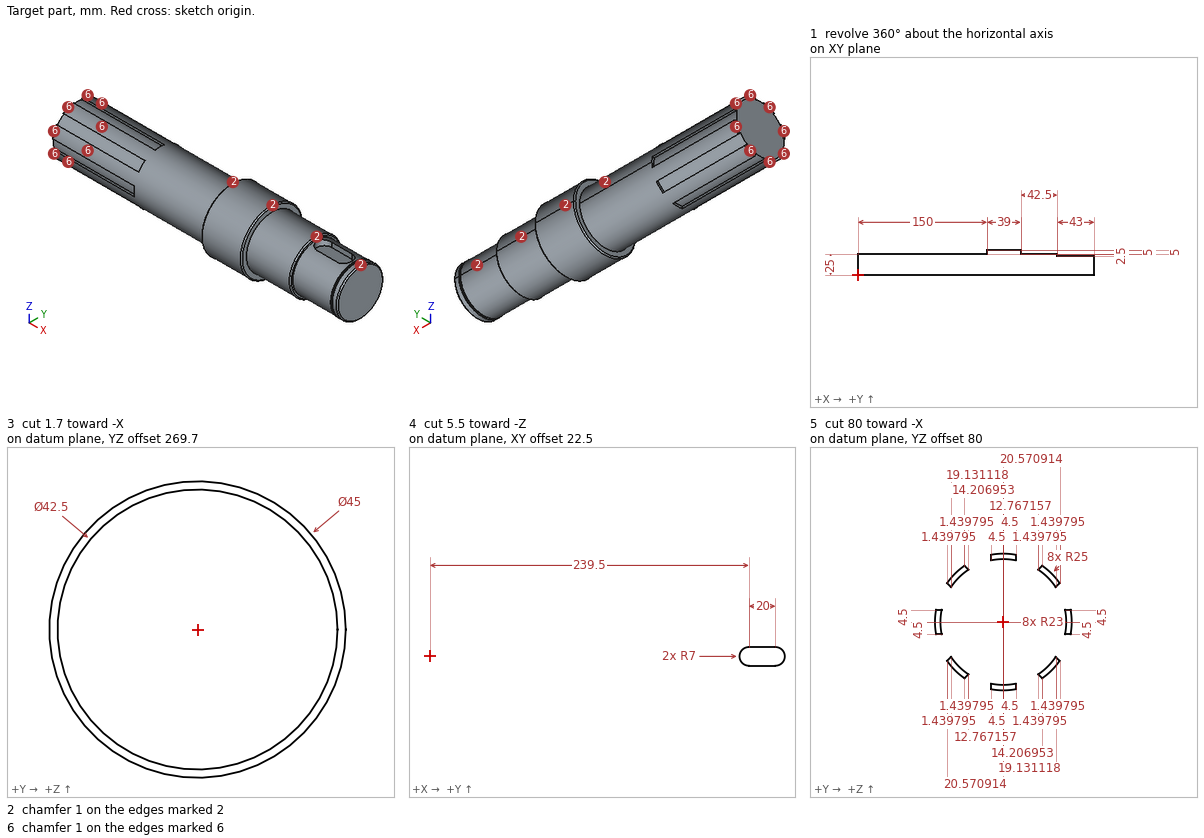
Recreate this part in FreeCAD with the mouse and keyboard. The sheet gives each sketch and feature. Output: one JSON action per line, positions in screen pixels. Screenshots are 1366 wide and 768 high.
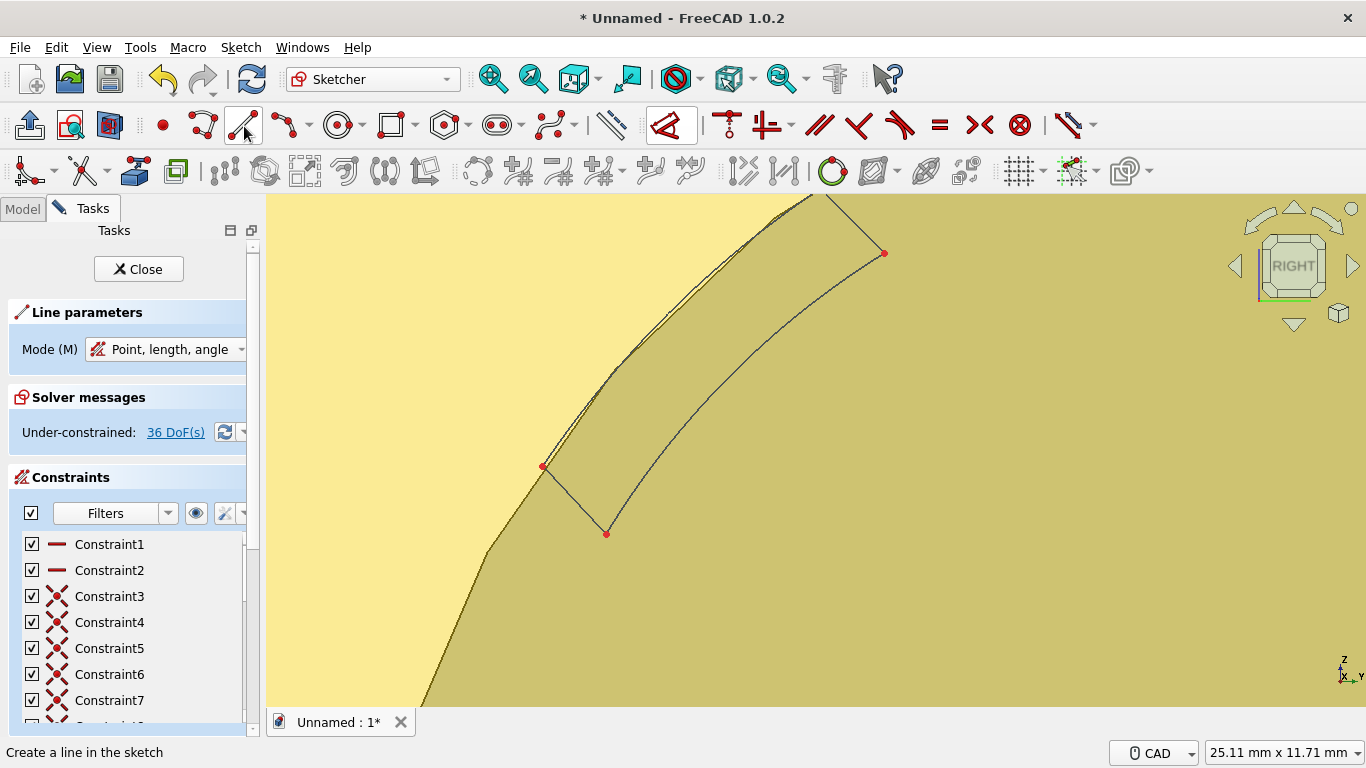
{"action": "scroll", "coordinate": [638, 351], "scroll_direction": "down", "scroll_amount": 10}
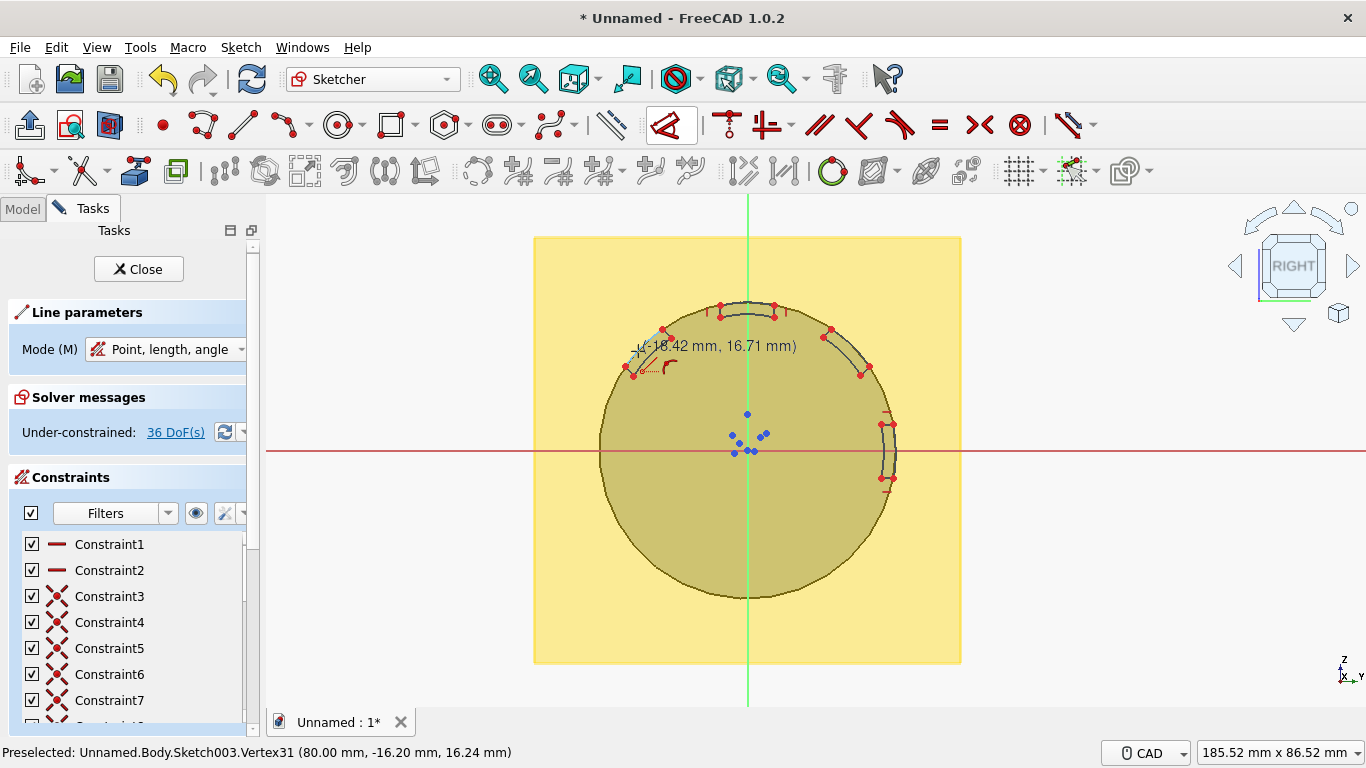
{"action": "left_click", "coordinate": [614, 477]}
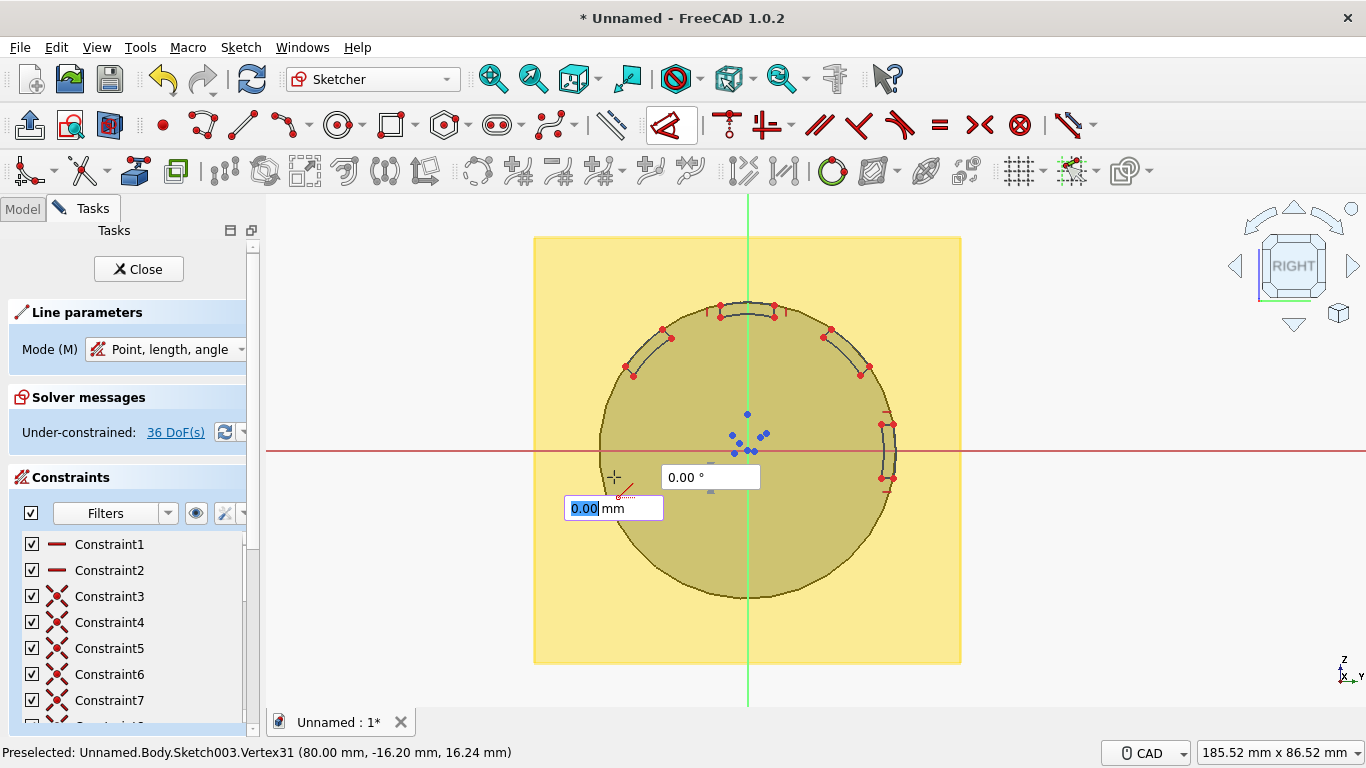
{"action": "scroll", "coordinate": [602, 477], "scroll_direction": "up", "scroll_amount": 2}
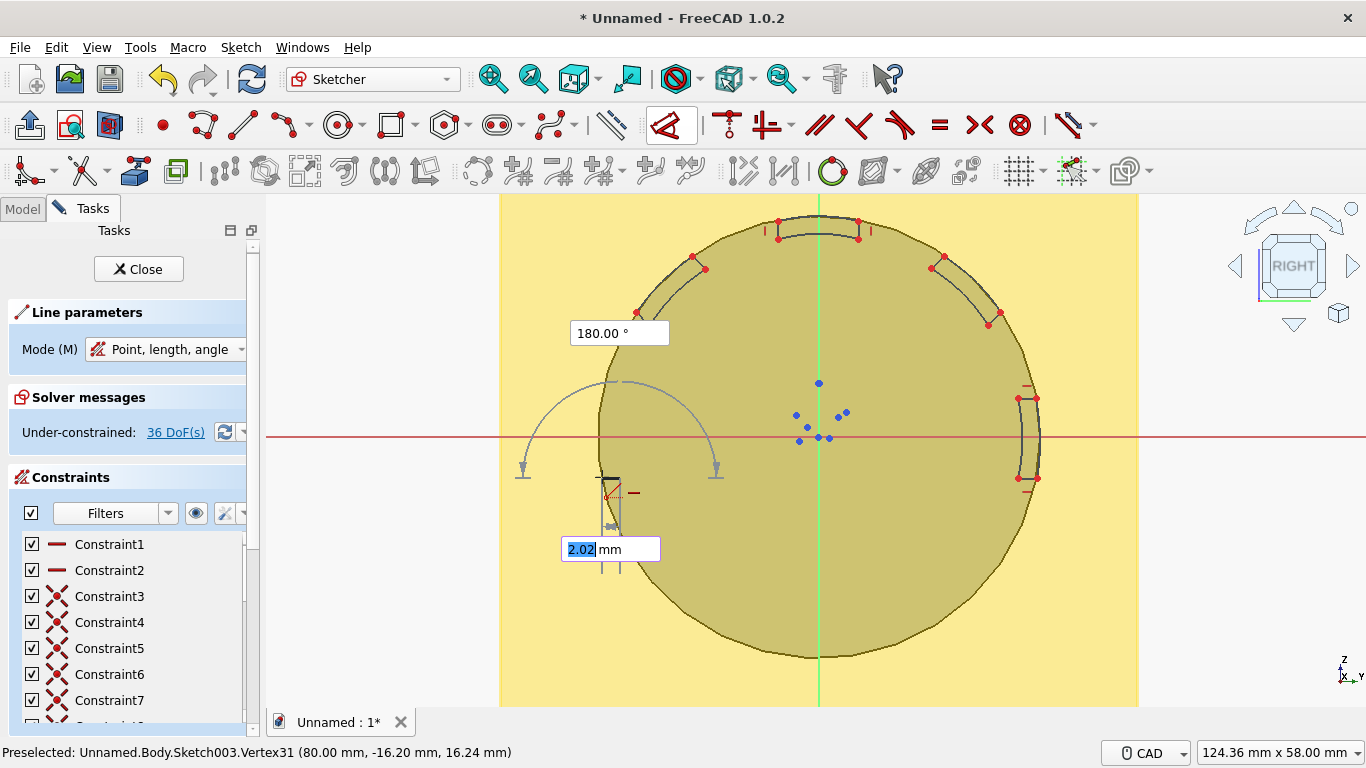
{"action": "left_click", "coordinate": [601, 477]}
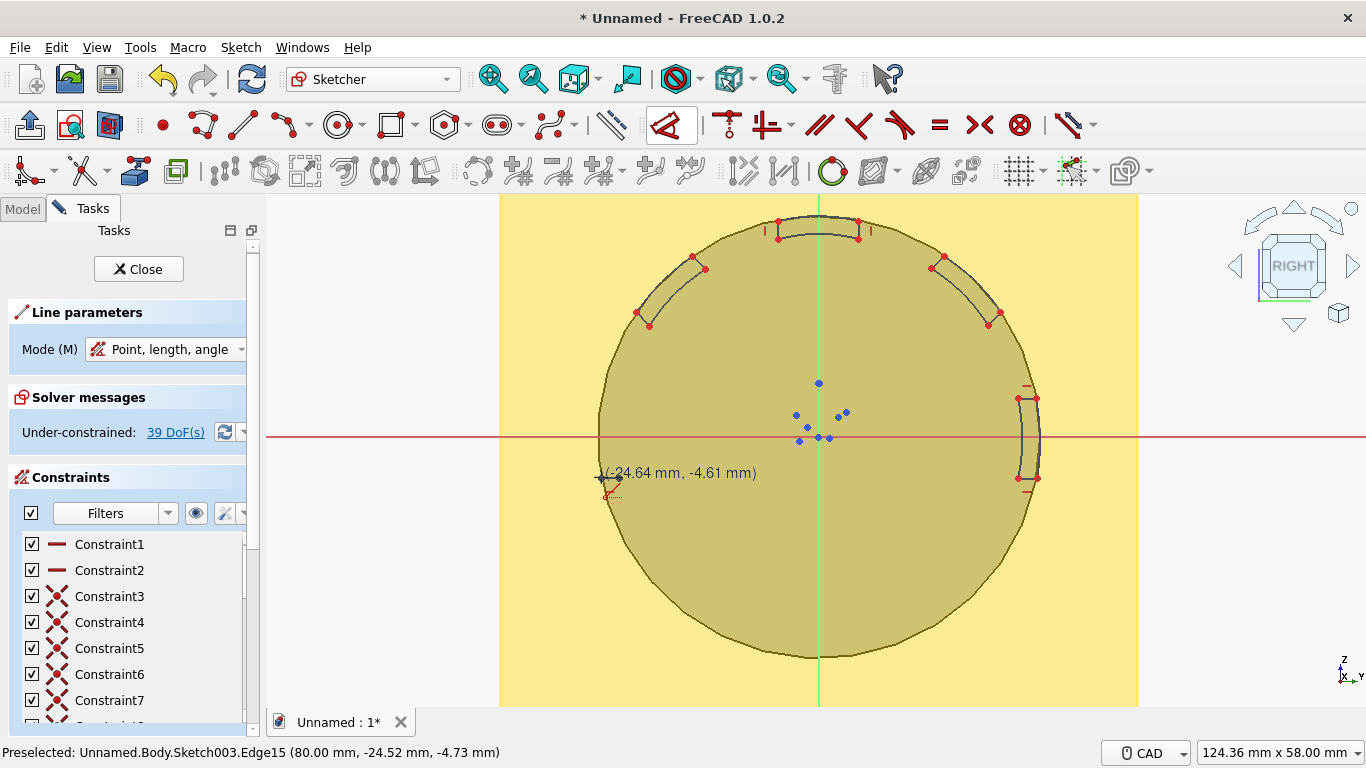
{"action": "left_click", "coordinate": [601, 397]}
{"action": "left_click", "coordinate": [619, 397]}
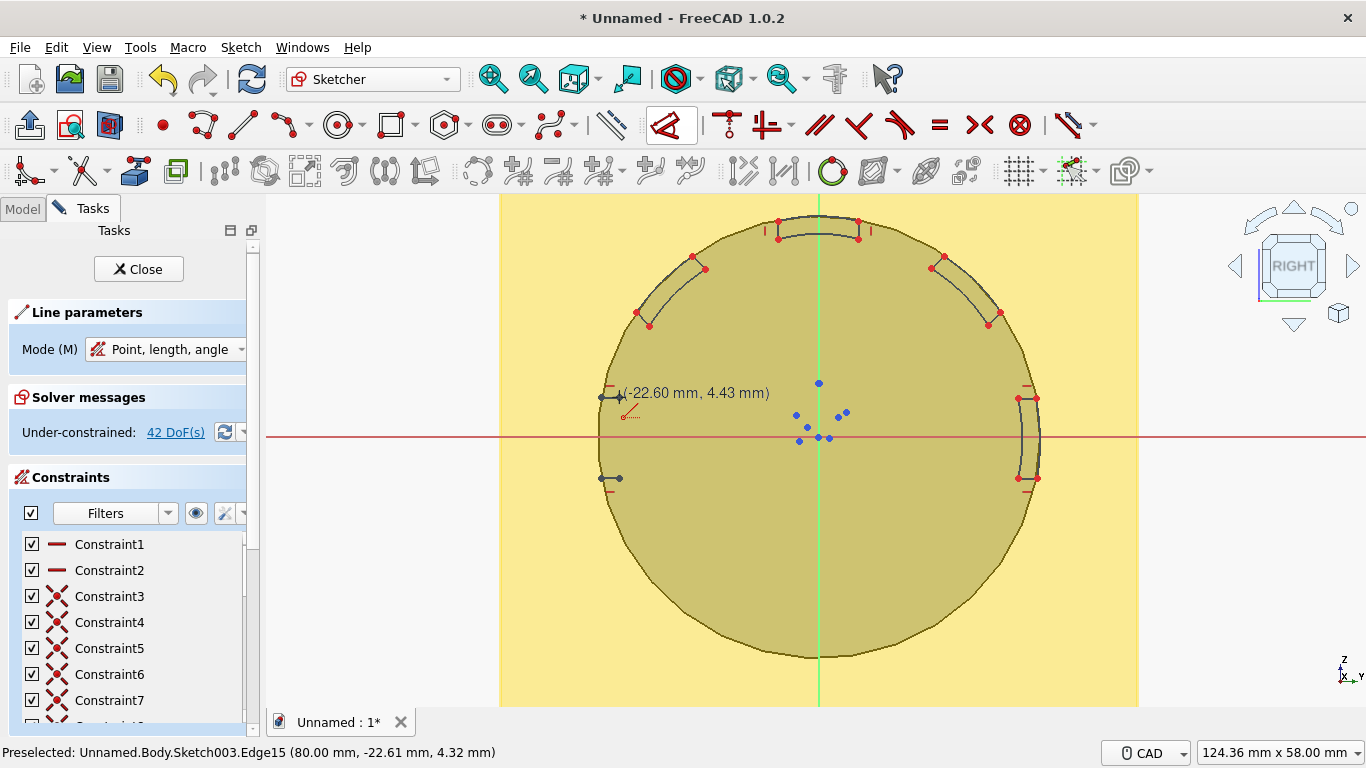
{"action": "key", "text": "g 3 a"}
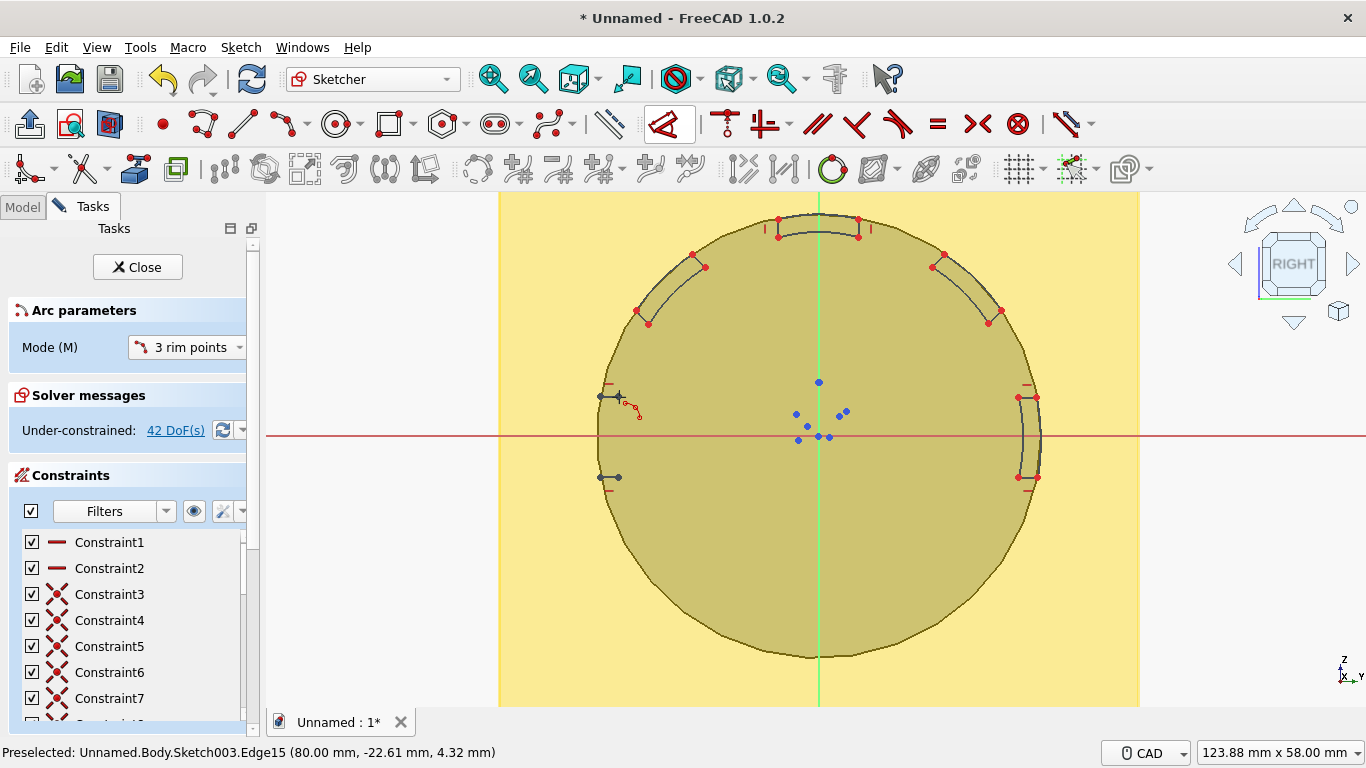
{"action": "scroll", "coordinate": [601, 476], "scroll_direction": "up", "scroll_amount": 3}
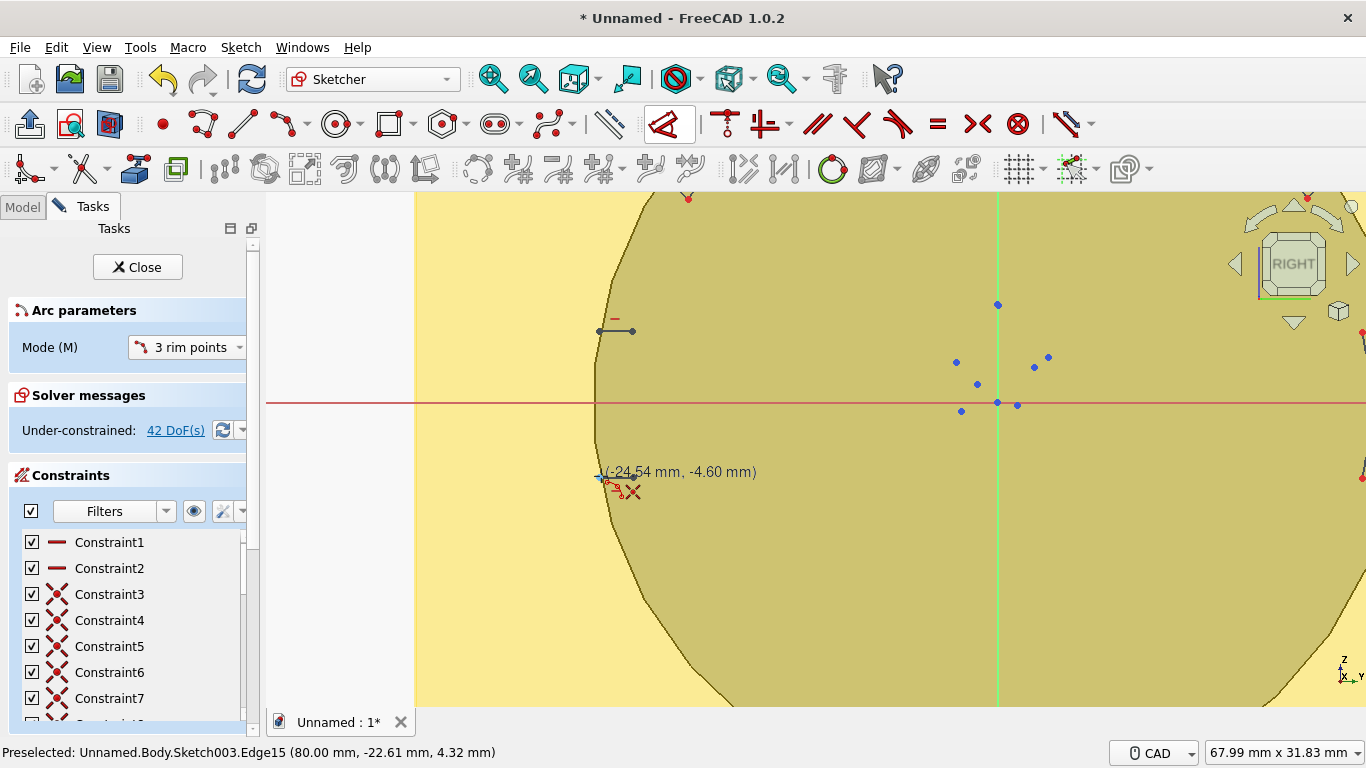
{"action": "left_click", "coordinate": [599, 478]}
{"action": "left_click", "coordinate": [599, 331]}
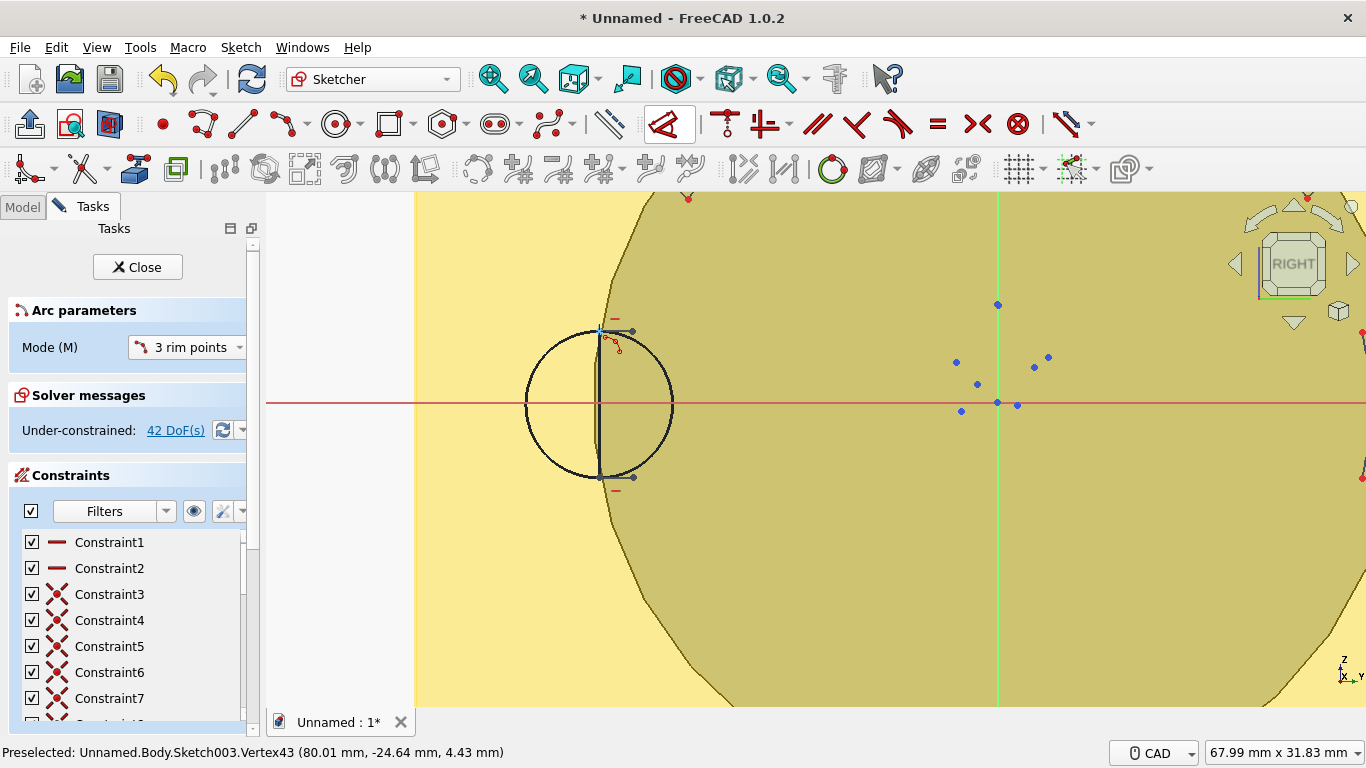
{"action": "scroll", "coordinate": [594, 388], "scroll_direction": "up", "scroll_amount": 5}